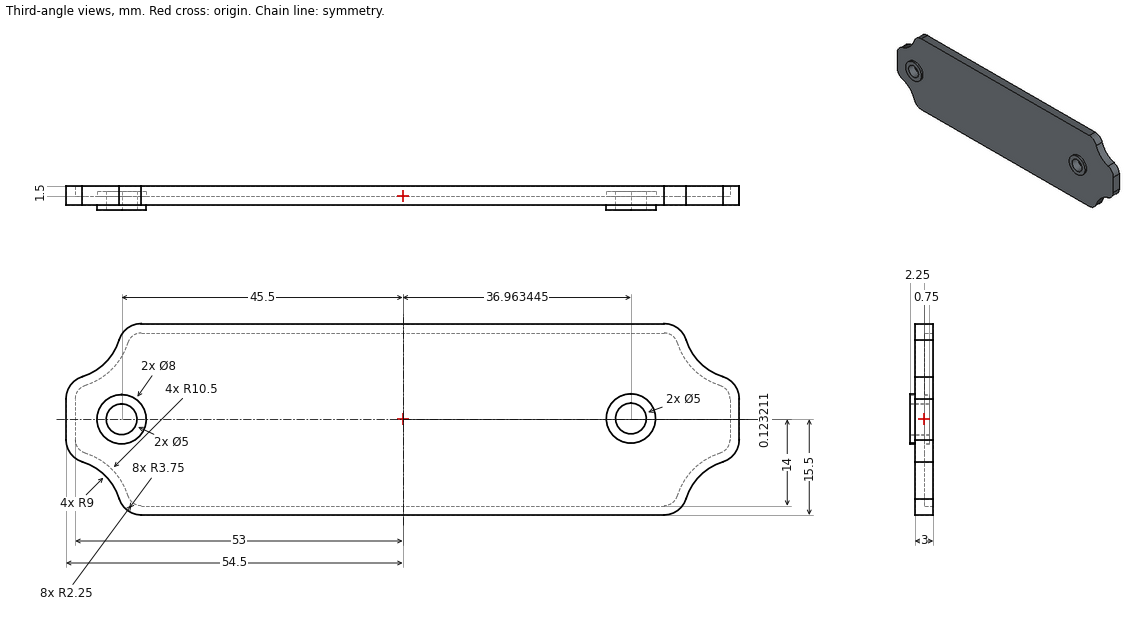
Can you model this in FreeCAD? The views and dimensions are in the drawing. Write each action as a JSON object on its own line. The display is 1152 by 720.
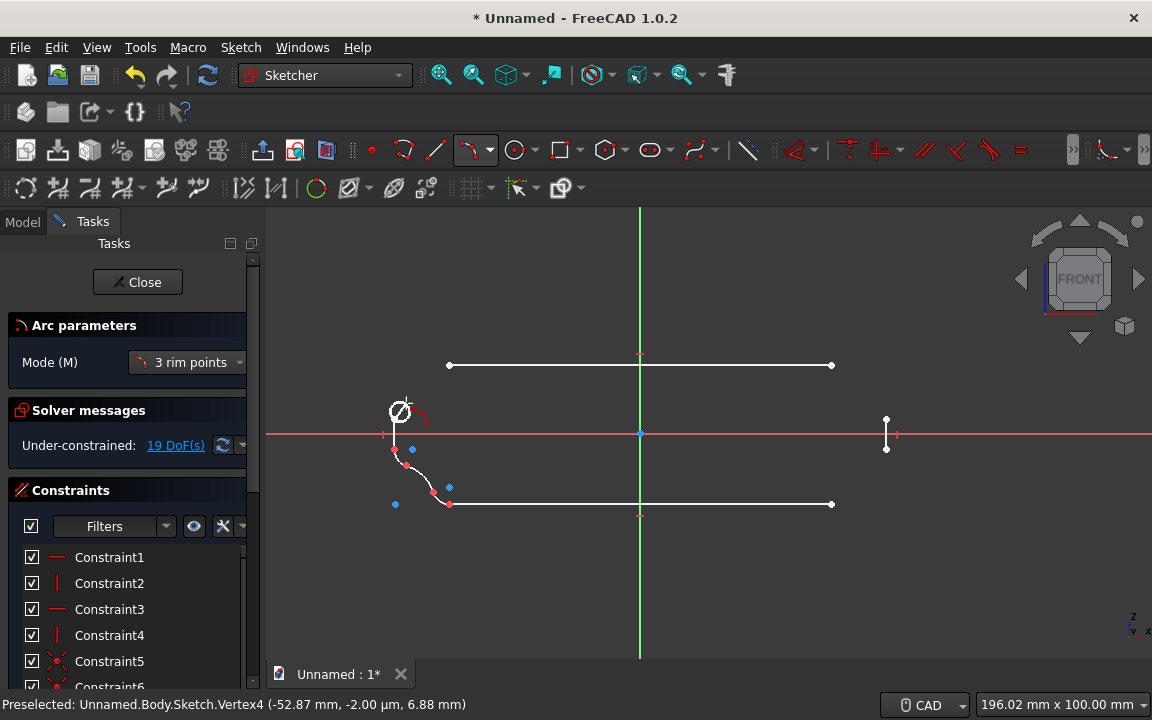
{"action": "scroll", "coordinate": [397, 409], "scroll_direction": "up", "scroll_amount": 8}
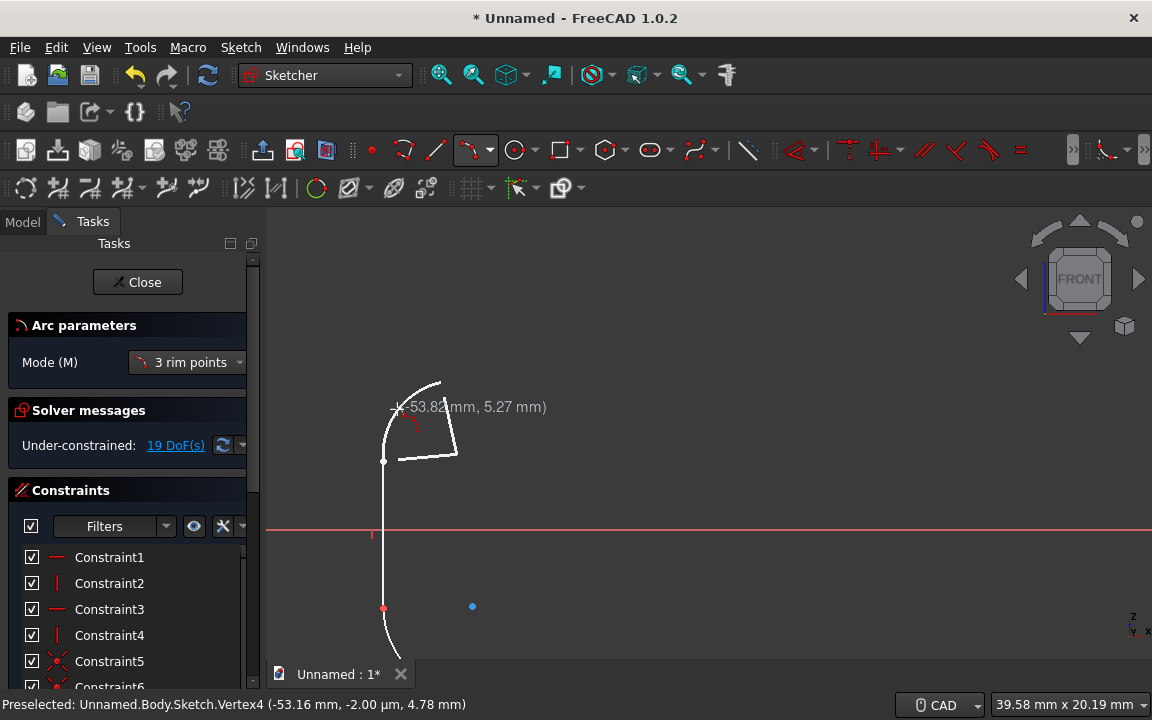
{"action": "left_click", "coordinate": [398, 406]}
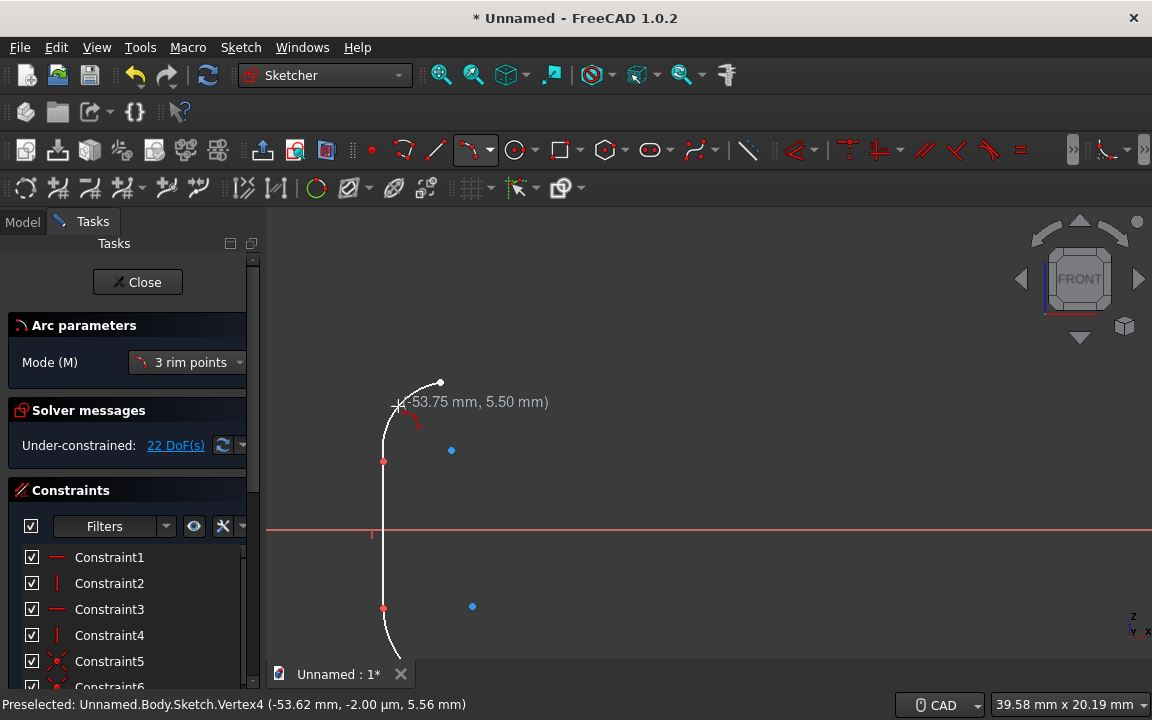
{"action": "scroll", "coordinate": [397, 408], "scroll_direction": "down", "scroll_amount": 8}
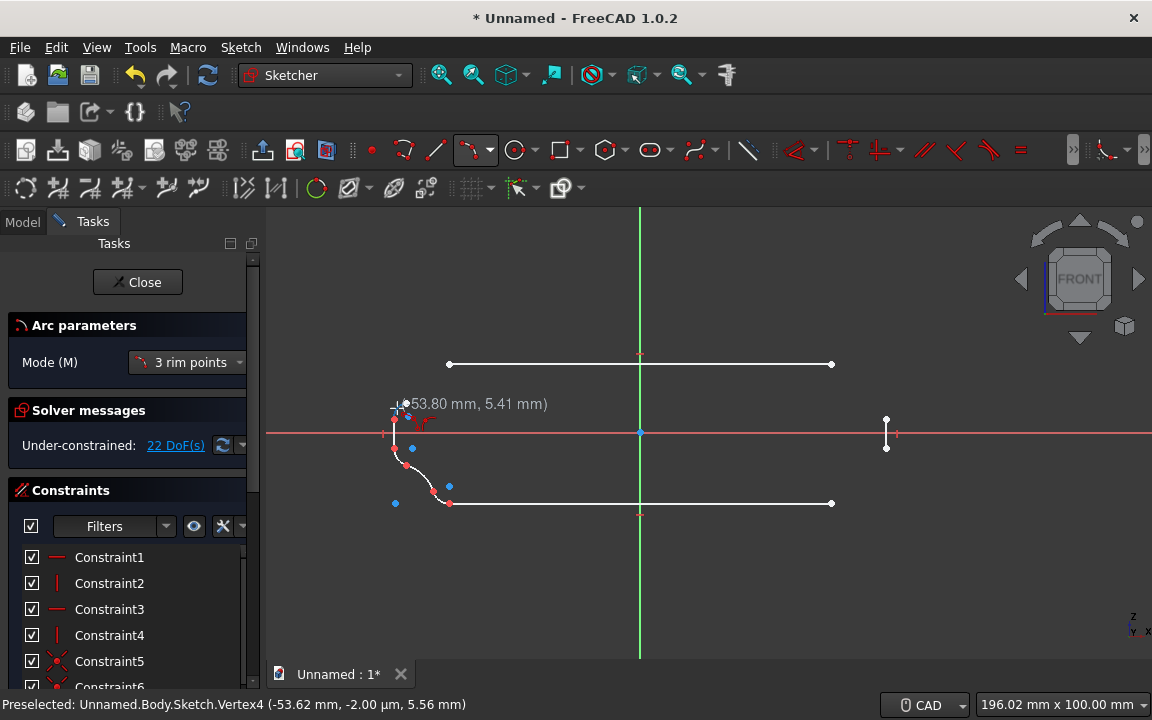
{"action": "left_click", "coordinate": [406, 403]}
{"action": "left_click", "coordinate": [433, 375]}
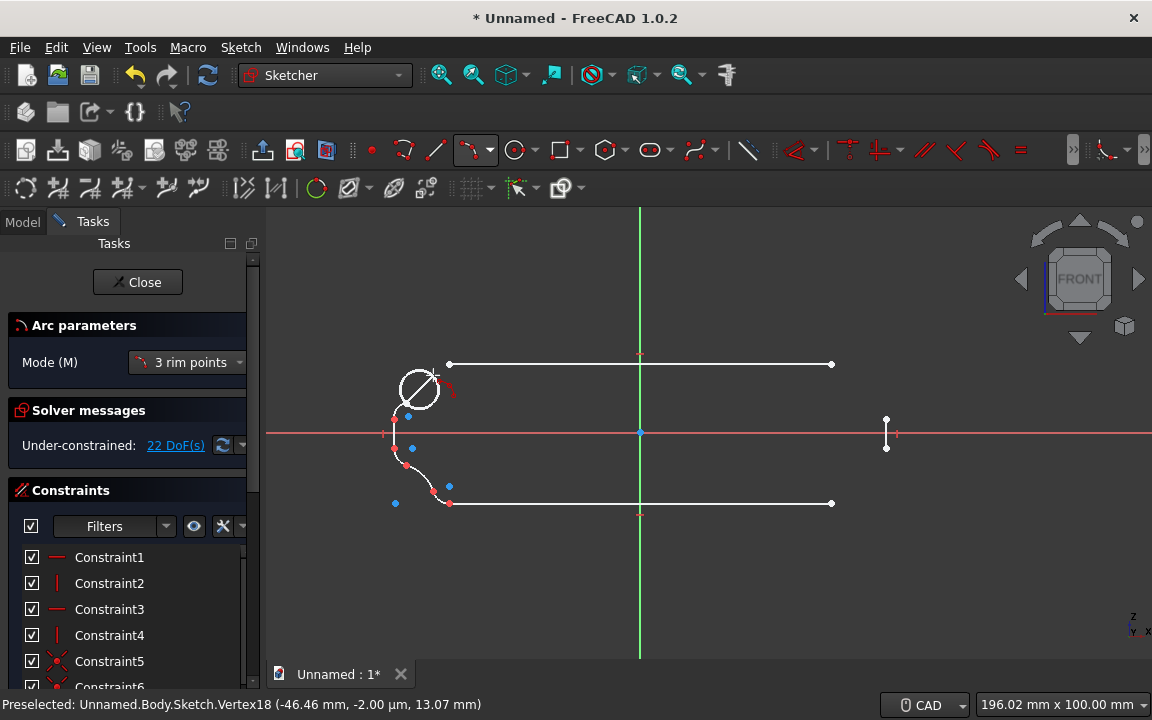
{"action": "scroll", "coordinate": [423, 392], "scroll_direction": "up", "scroll_amount": 7}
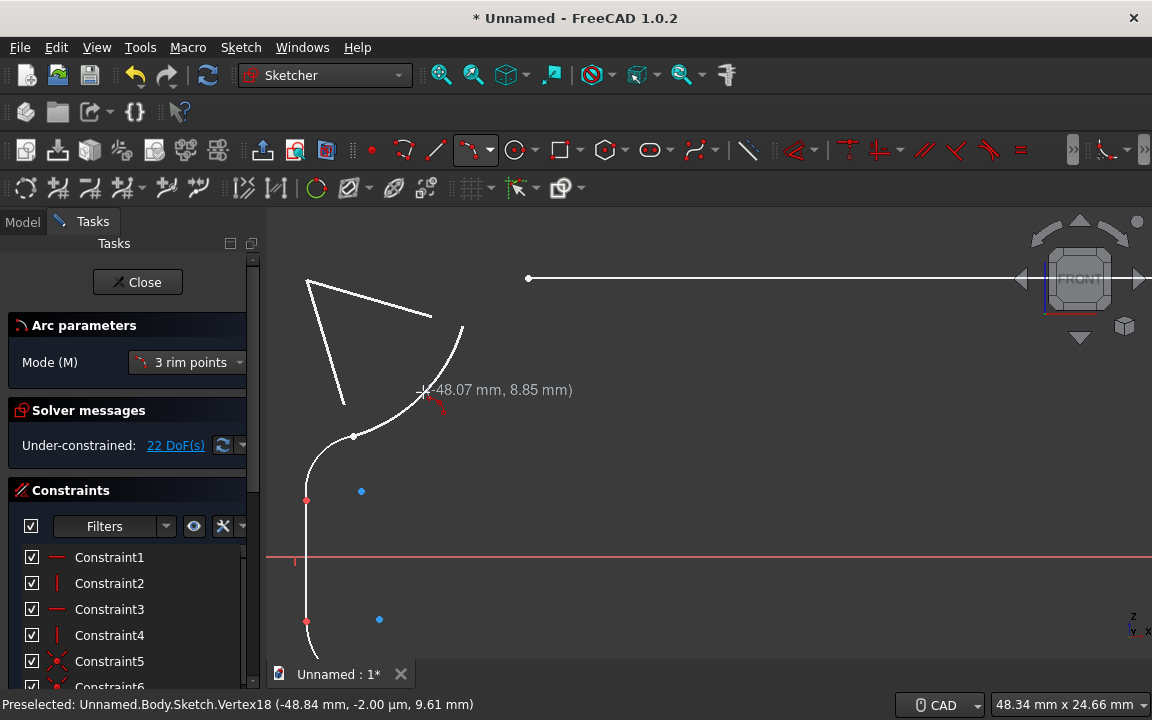
{"action": "left_click", "coordinate": [421, 390]}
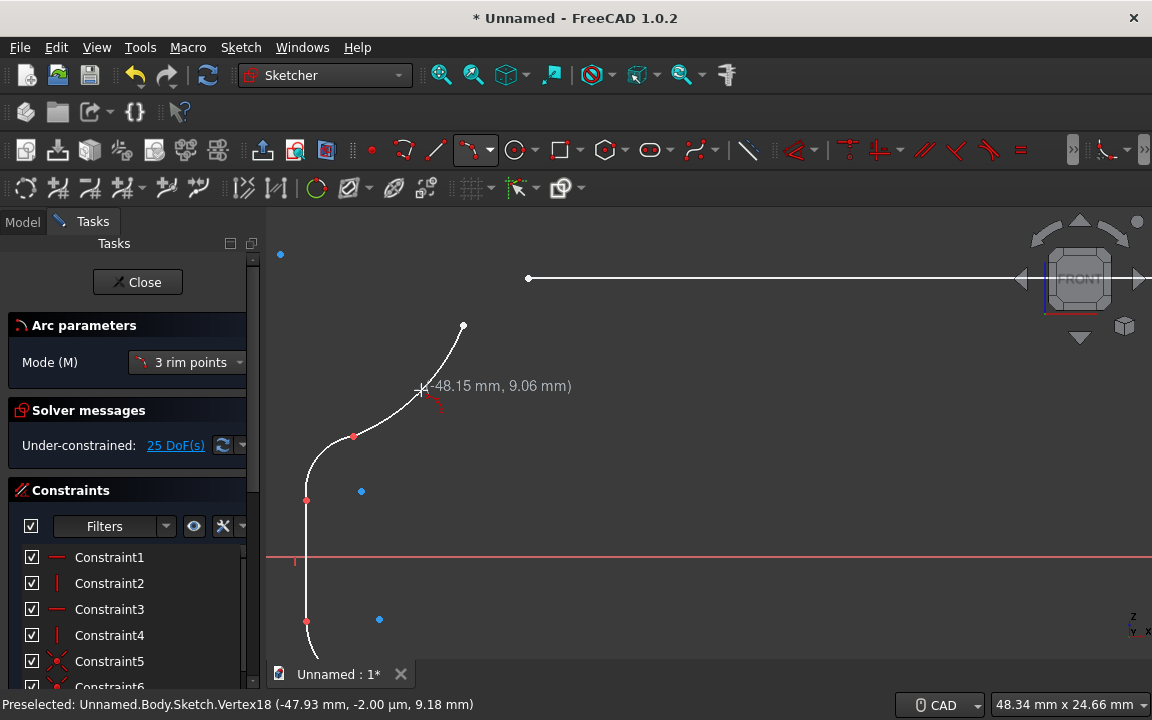
{"action": "scroll", "coordinate": [423, 392], "scroll_direction": "down", "scroll_amount": 7}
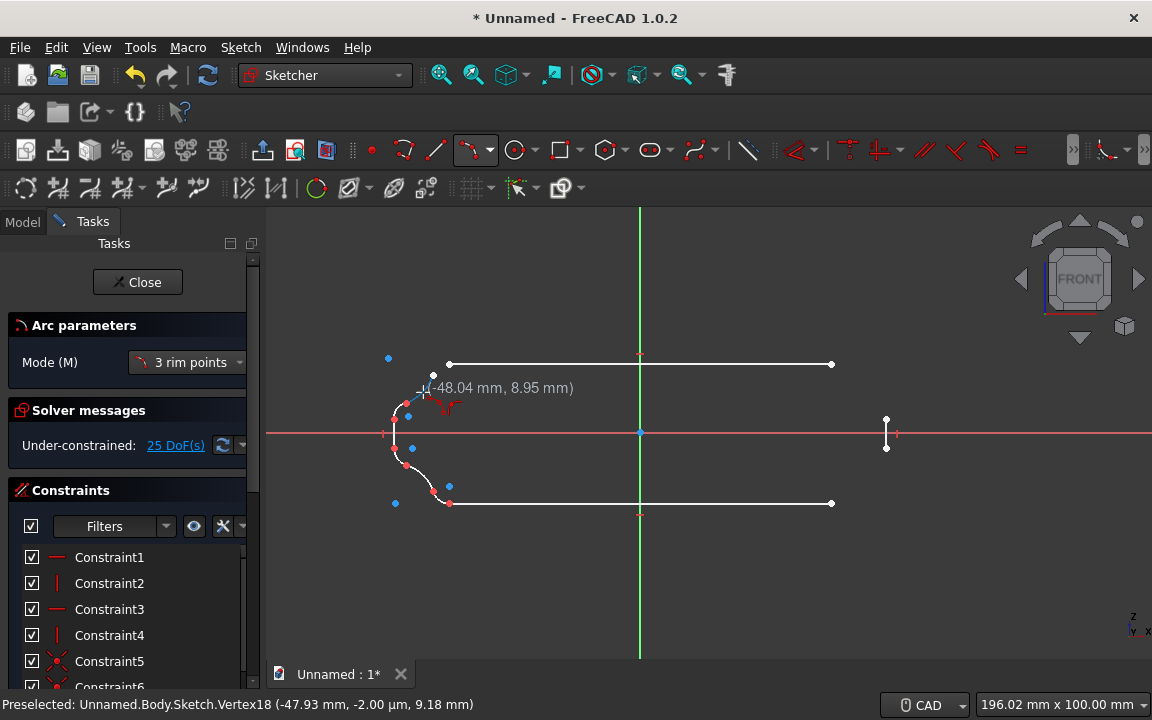
{"action": "left_click", "coordinate": [433, 376]}
{"action": "left_click", "coordinate": [449, 364]}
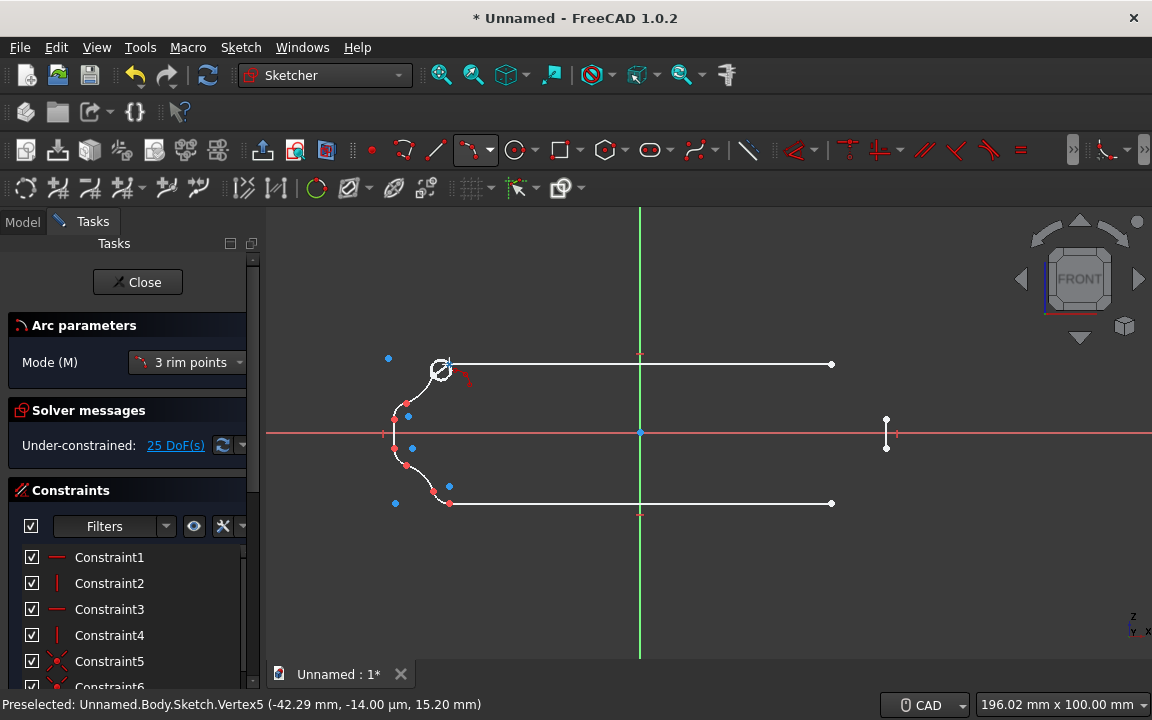
{"action": "scroll", "coordinate": [439, 366], "scroll_direction": "up", "scroll_amount": 8}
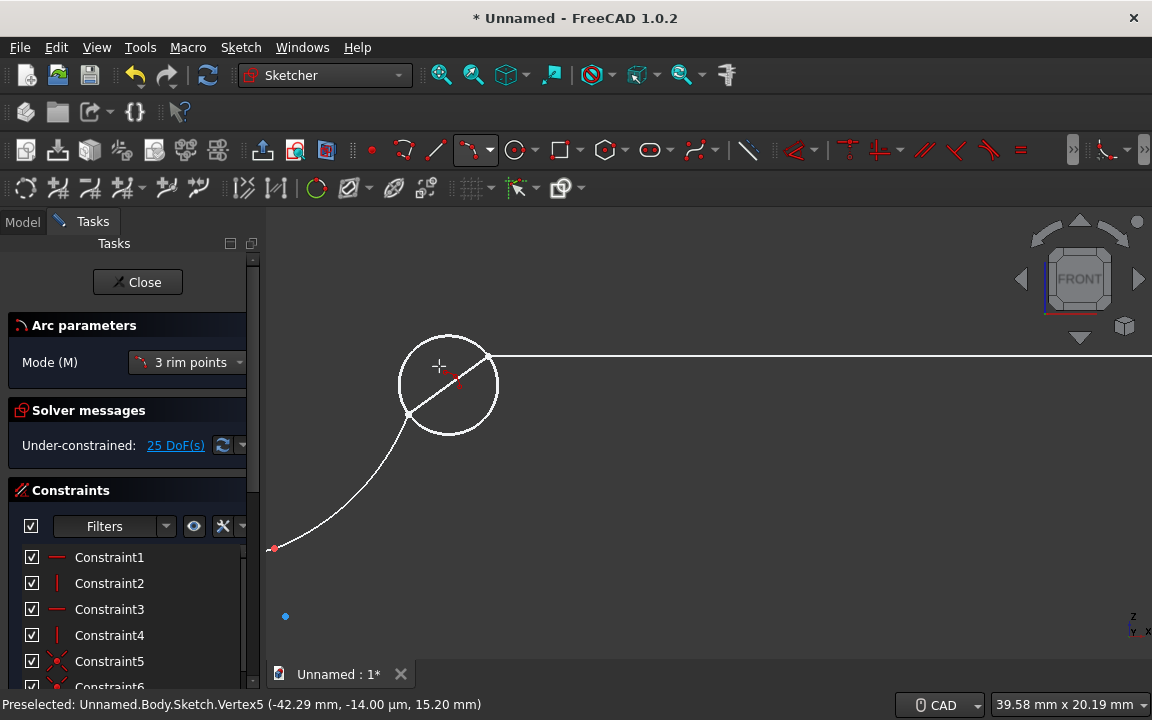
{"action": "left_click", "coordinate": [438, 366]}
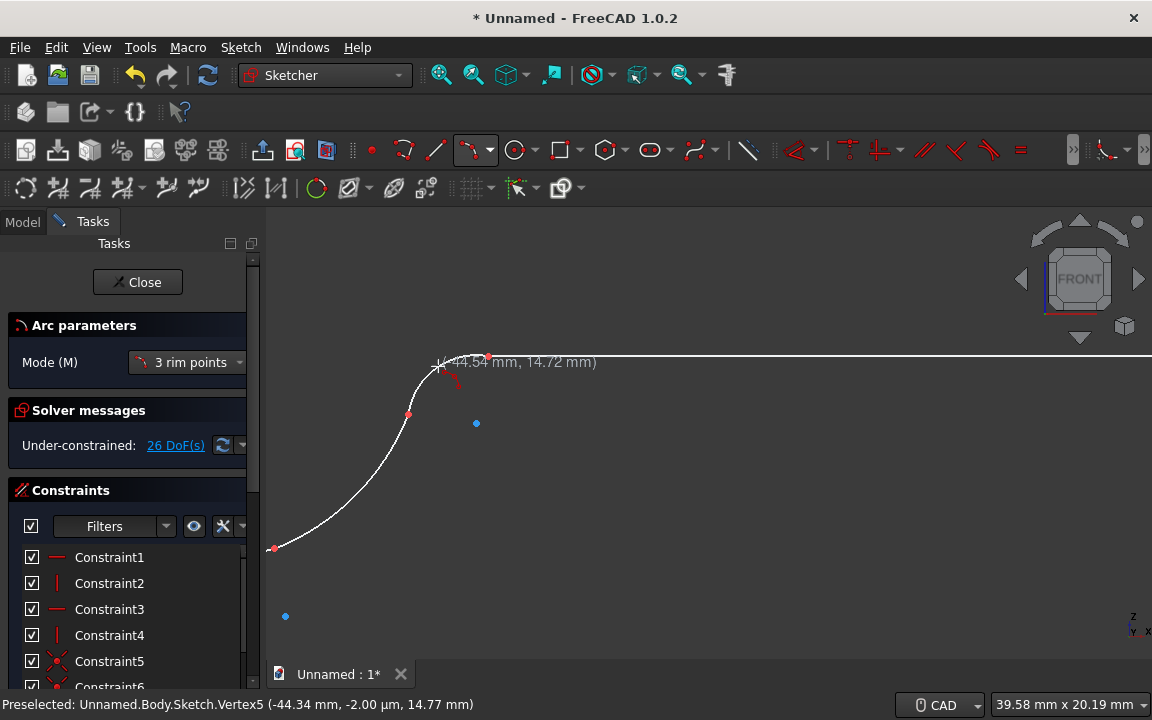
{"action": "scroll", "coordinate": [439, 366], "scroll_direction": "down", "scroll_amount": 8}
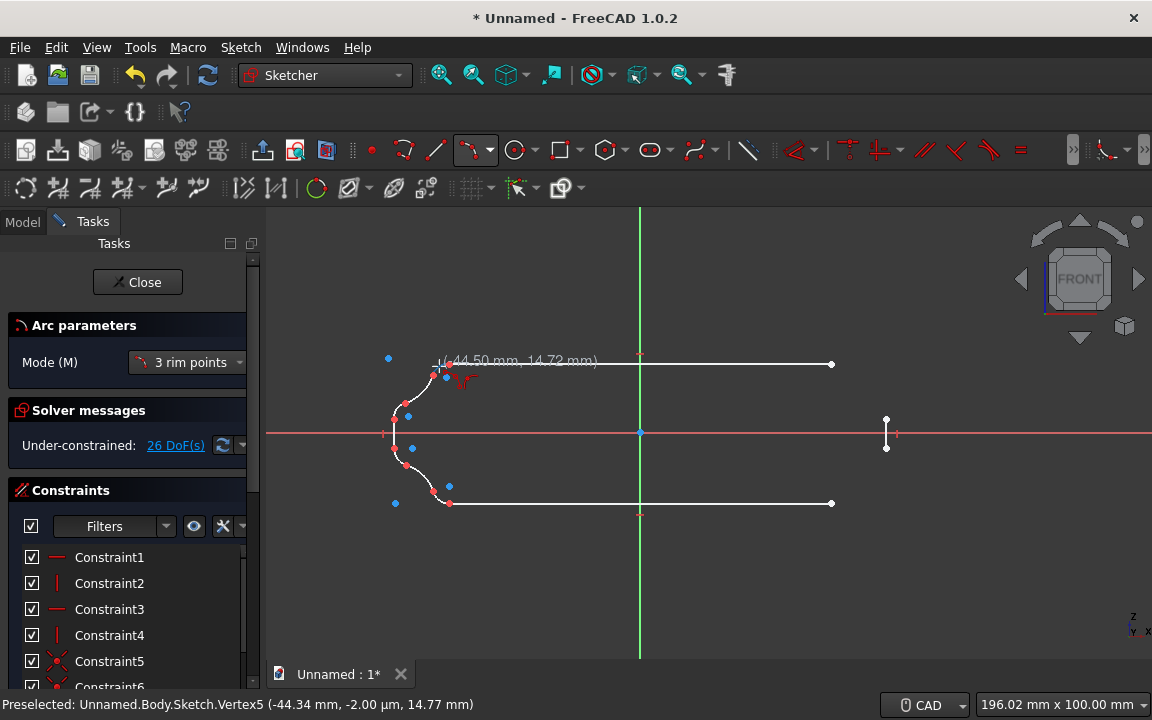
{"action": "left_click", "coordinate": [831, 364]}
{"action": "left_click", "coordinate": [848, 375]}